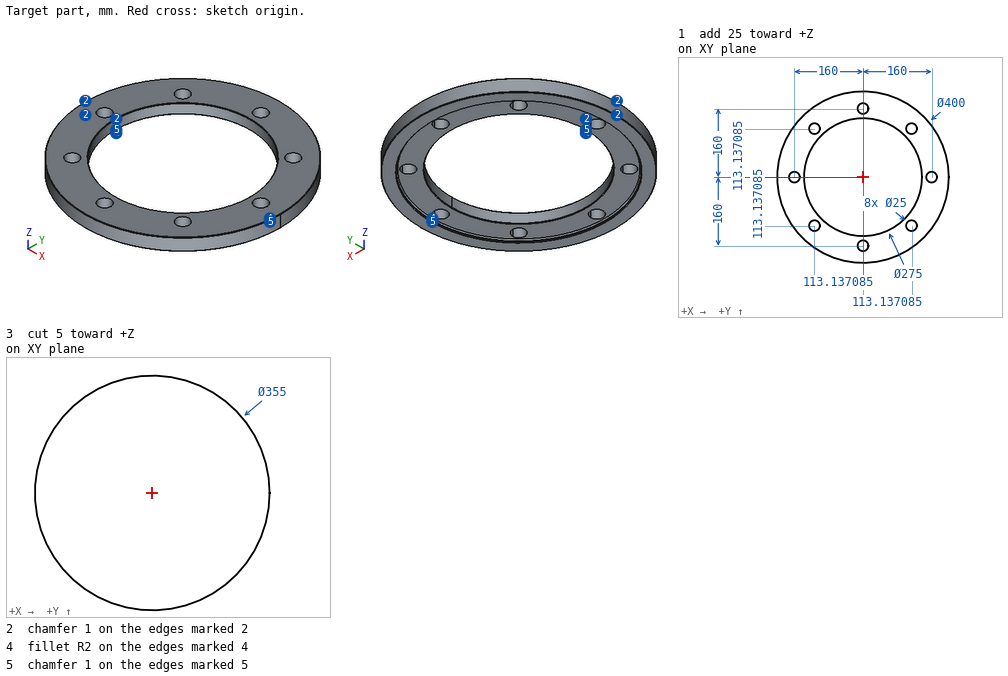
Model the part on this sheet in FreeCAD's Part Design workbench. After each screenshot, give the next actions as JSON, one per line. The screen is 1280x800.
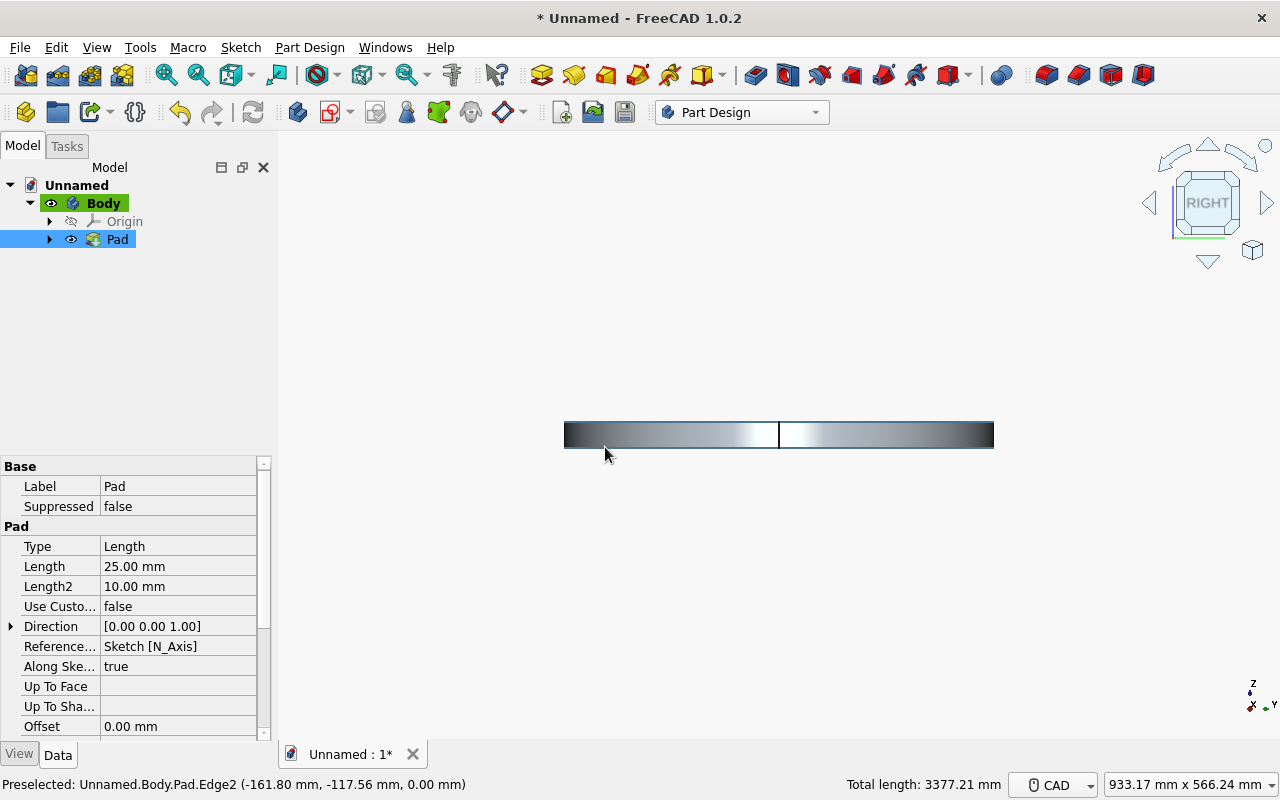
{"action": "left_click", "coordinate": [168, 76]}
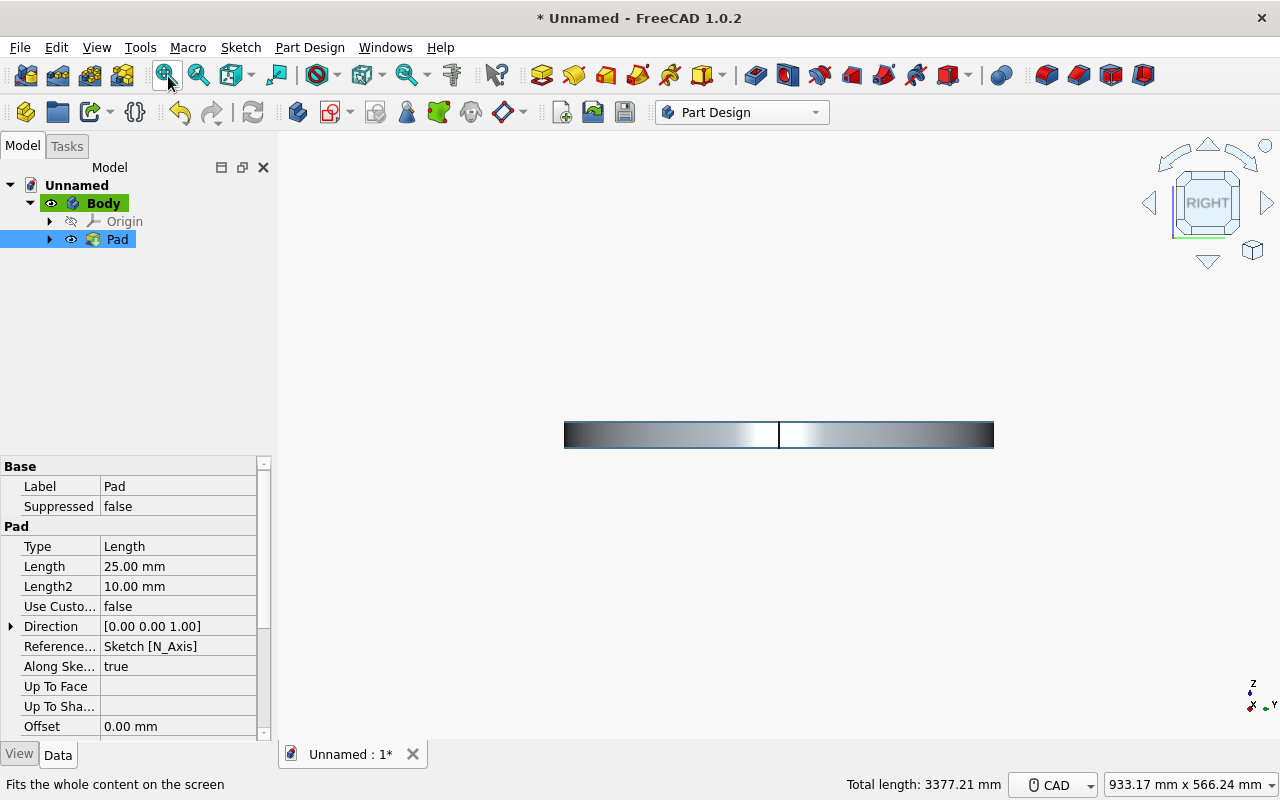
{"action": "key", "text": "5"}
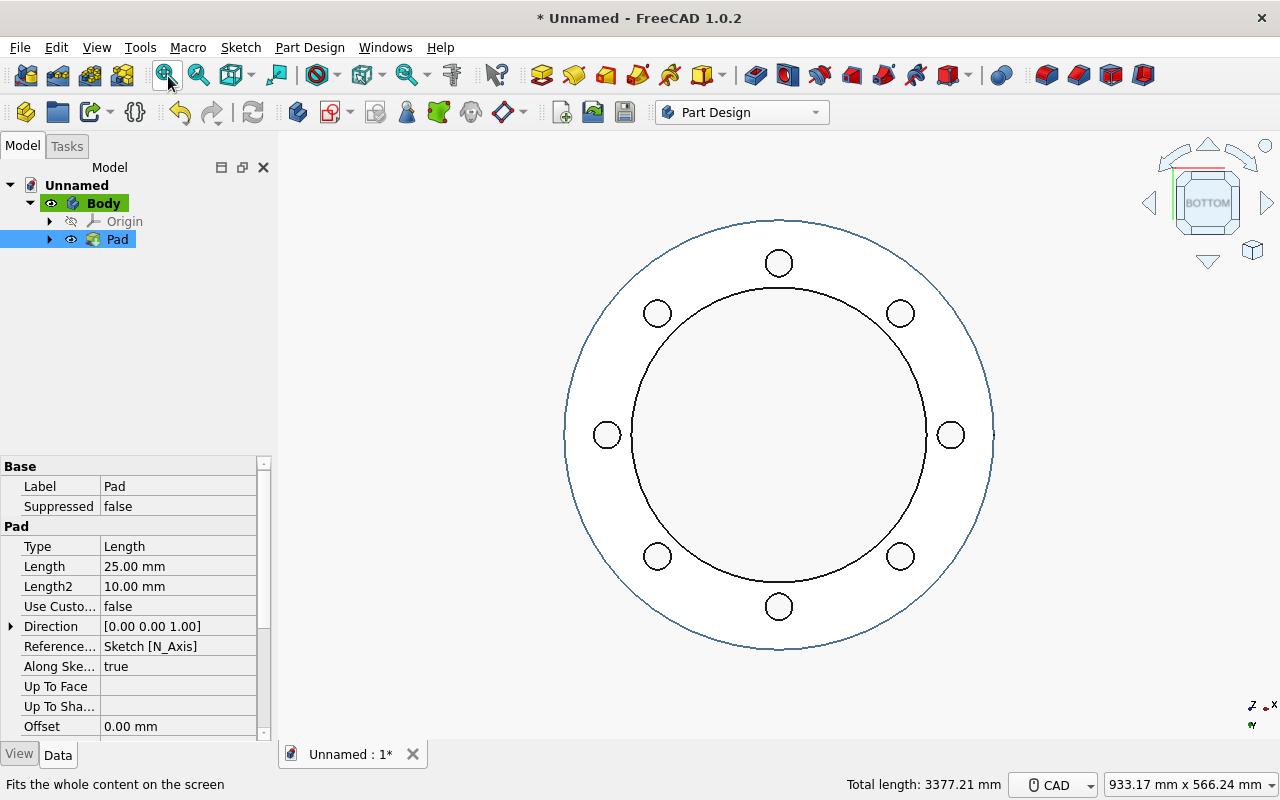
{"action": "left_click", "coordinate": [631, 434], "text": "ctrl"}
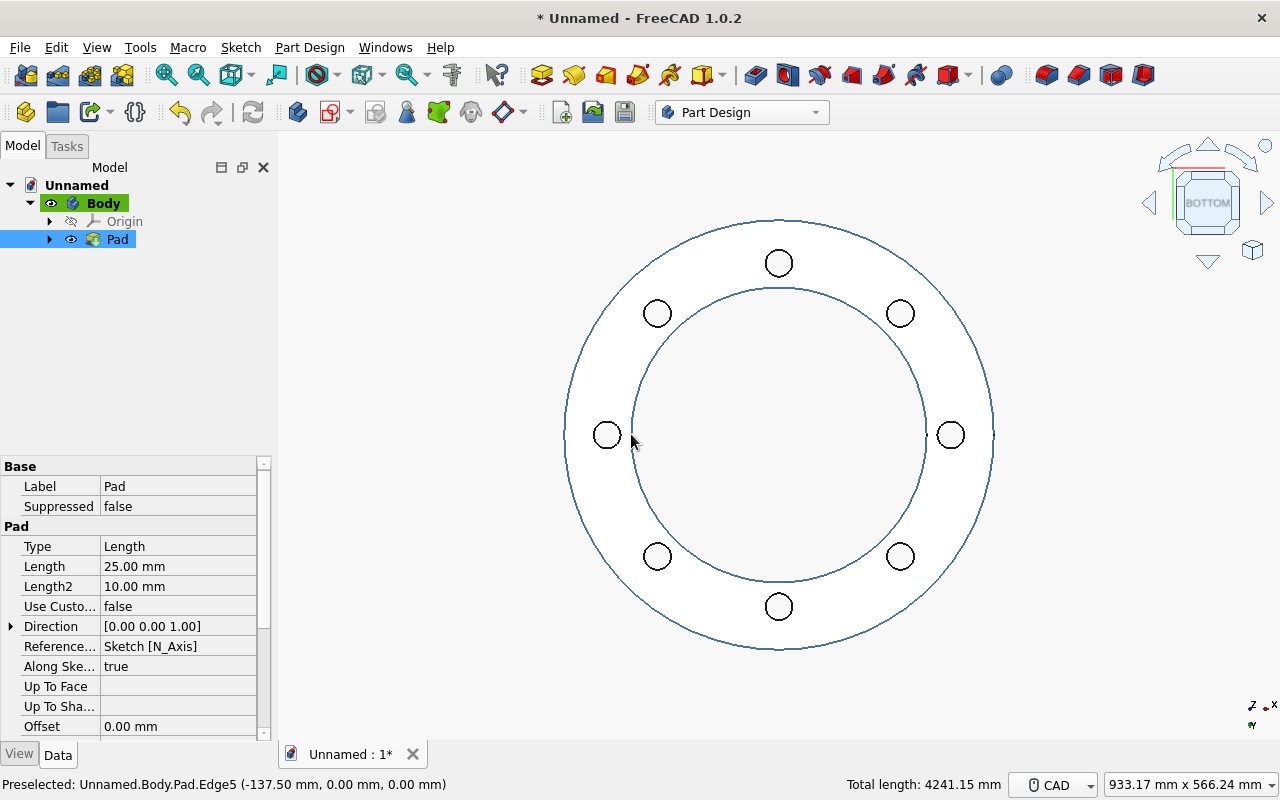
{"action": "left_click", "coordinate": [1080, 76]}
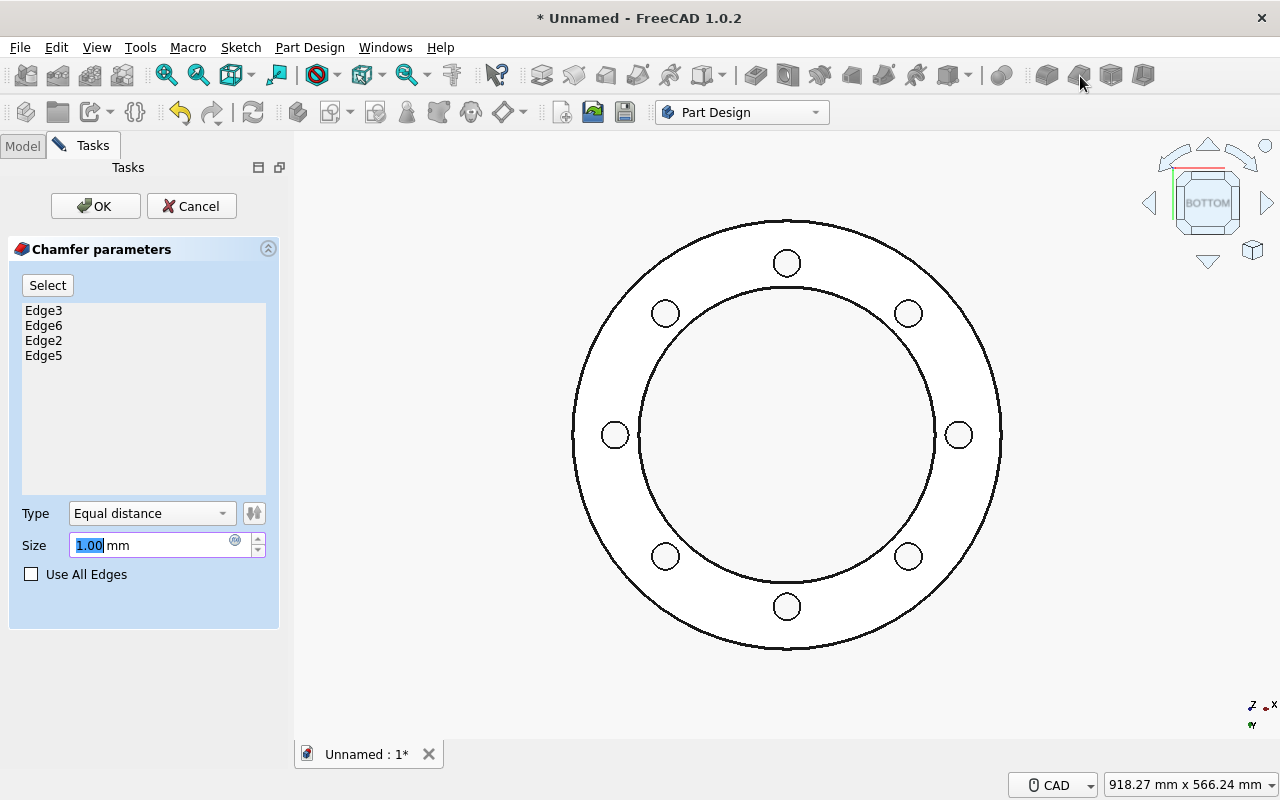
{"action": "type", "text": "1"}
{"action": "key", "text": "Tab"}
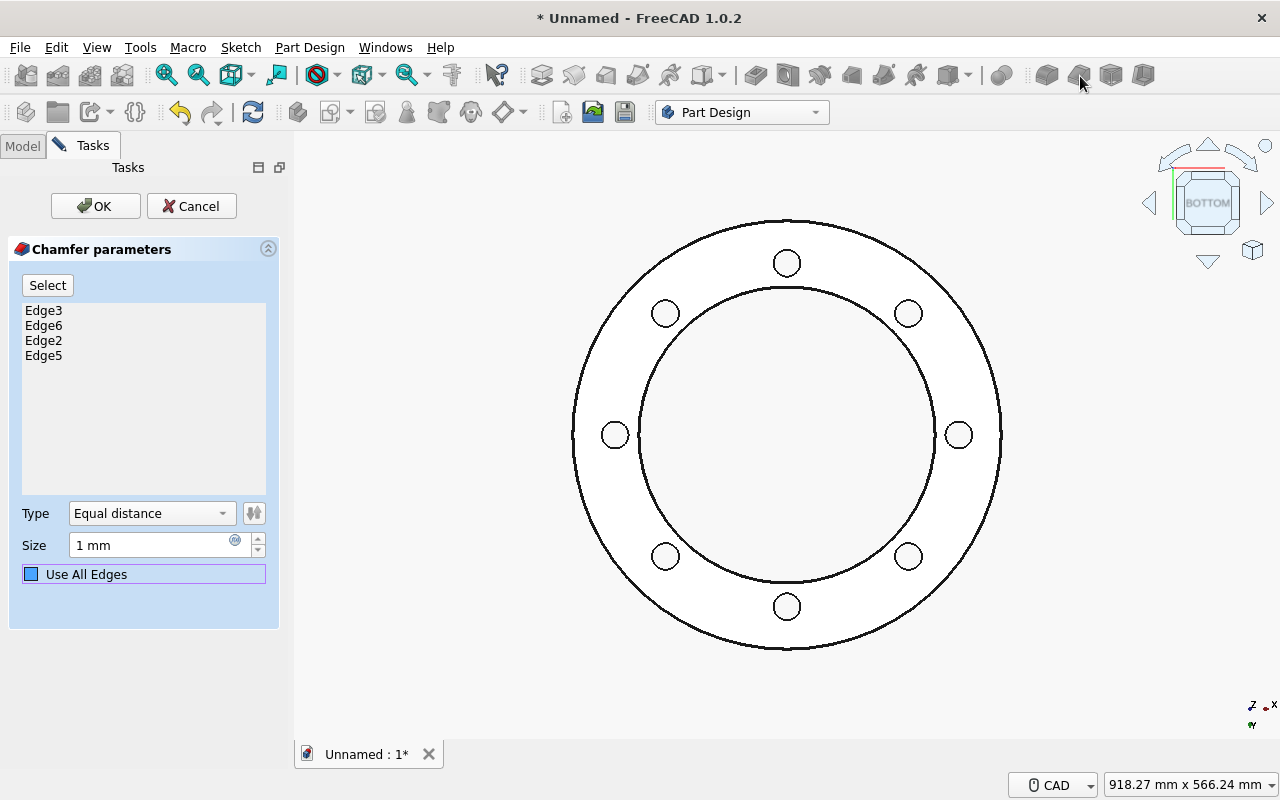
{"action": "left_click", "coordinate": [96, 206]}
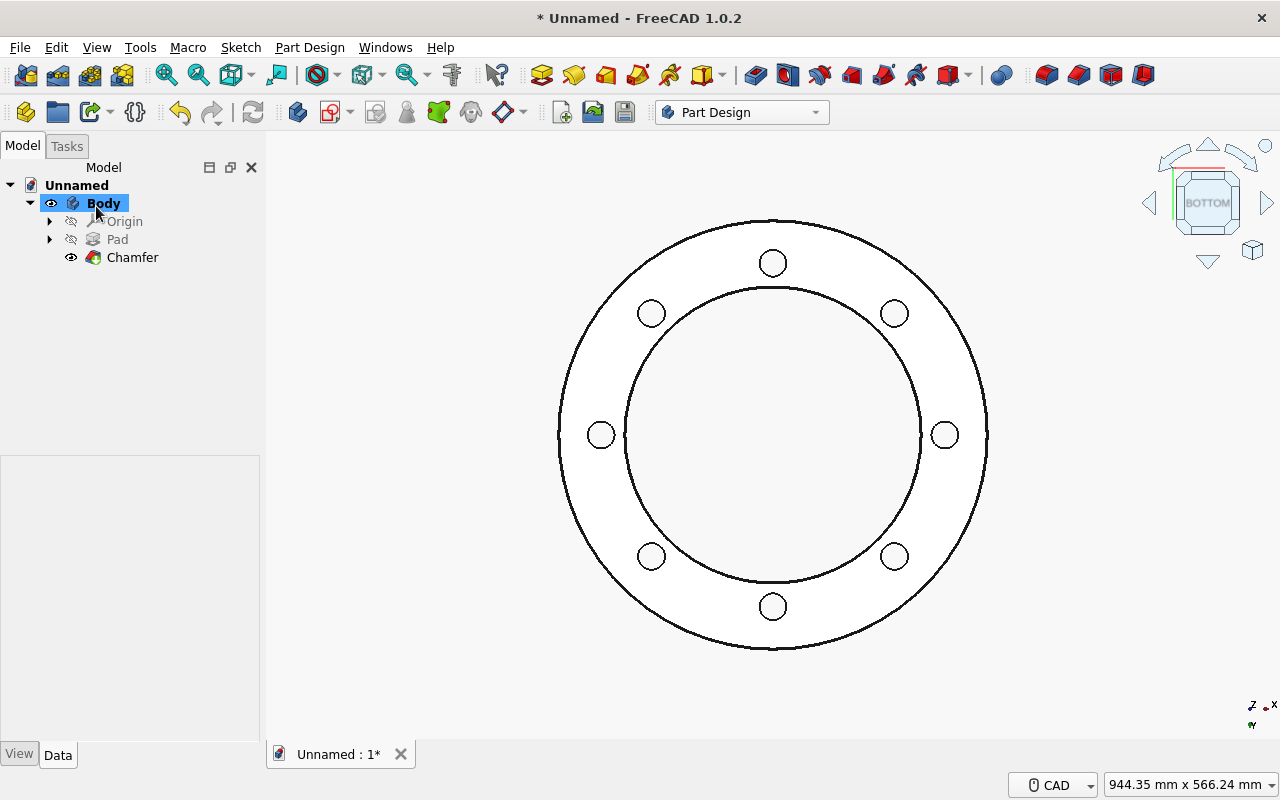
{"action": "left_click", "coordinate": [330, 112]}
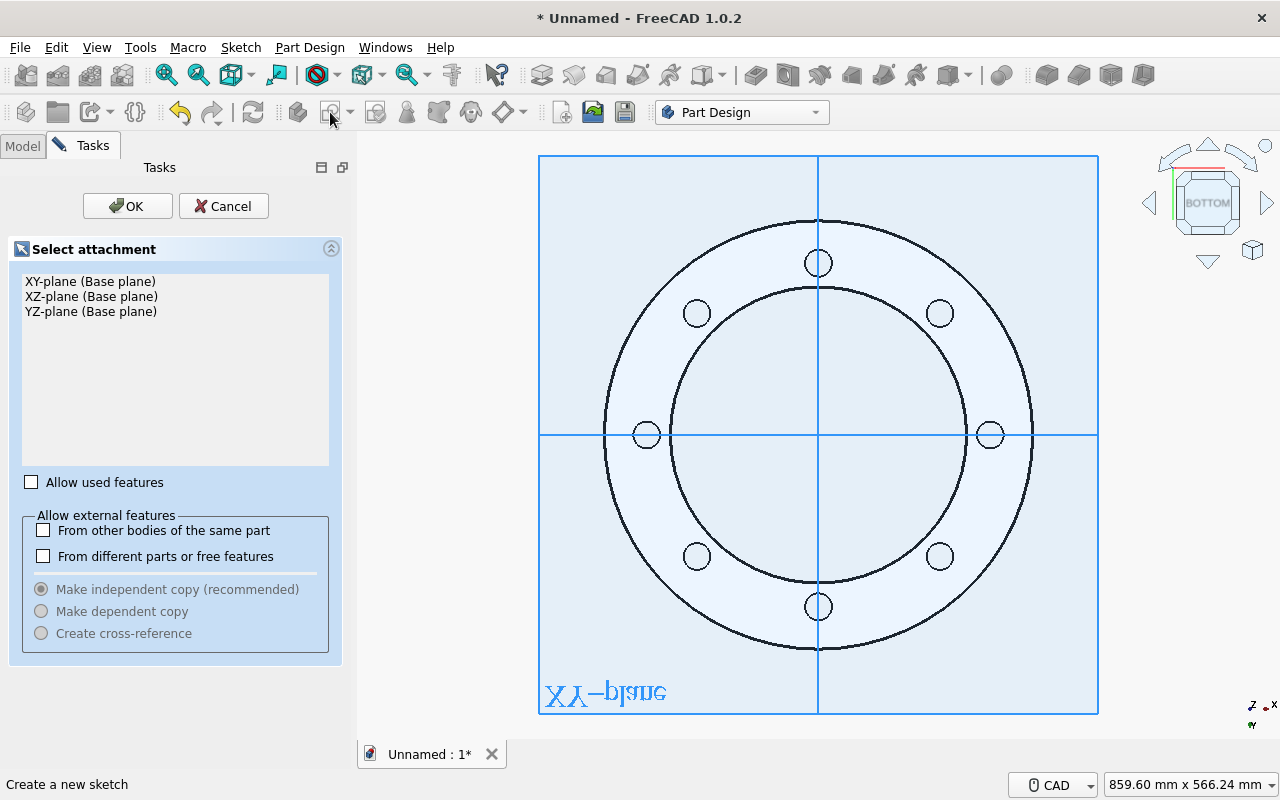
{"action": "left_click", "coordinate": [82, 282]}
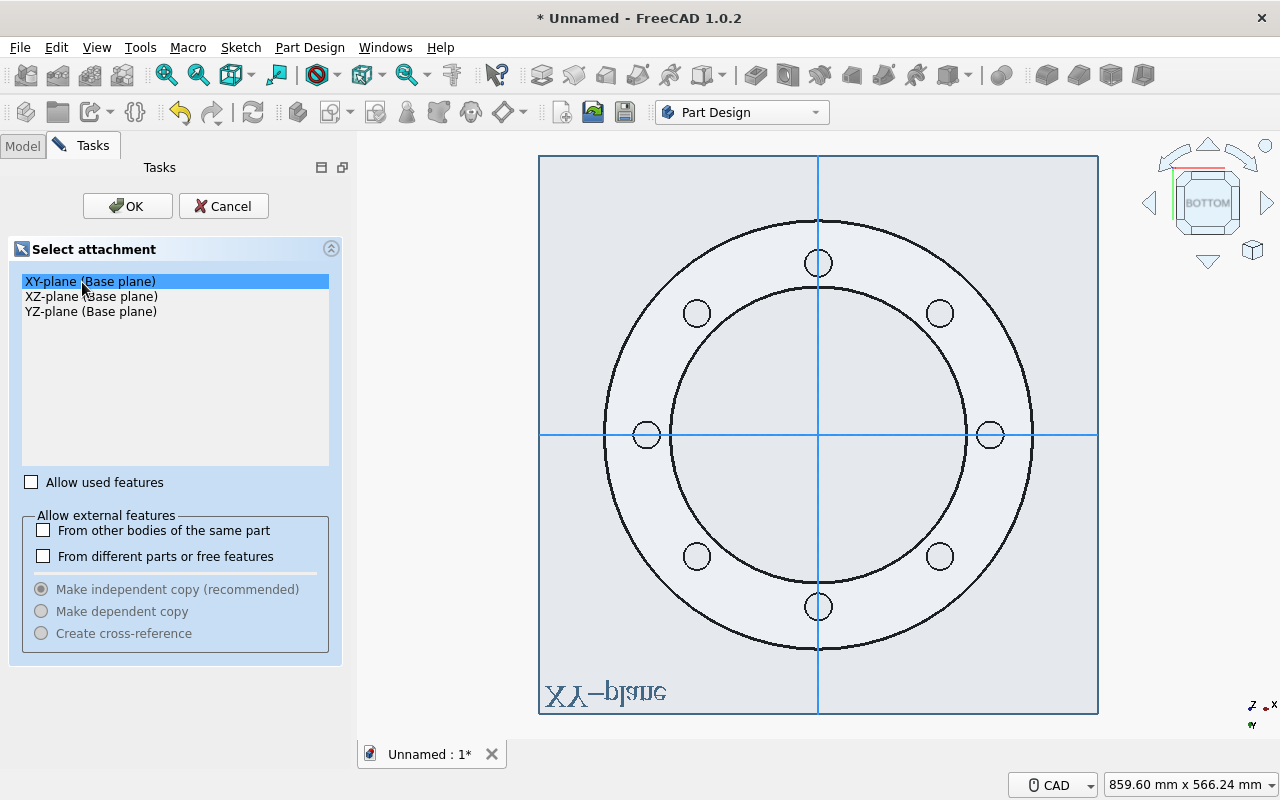
{"action": "left_click", "coordinate": [128, 206]}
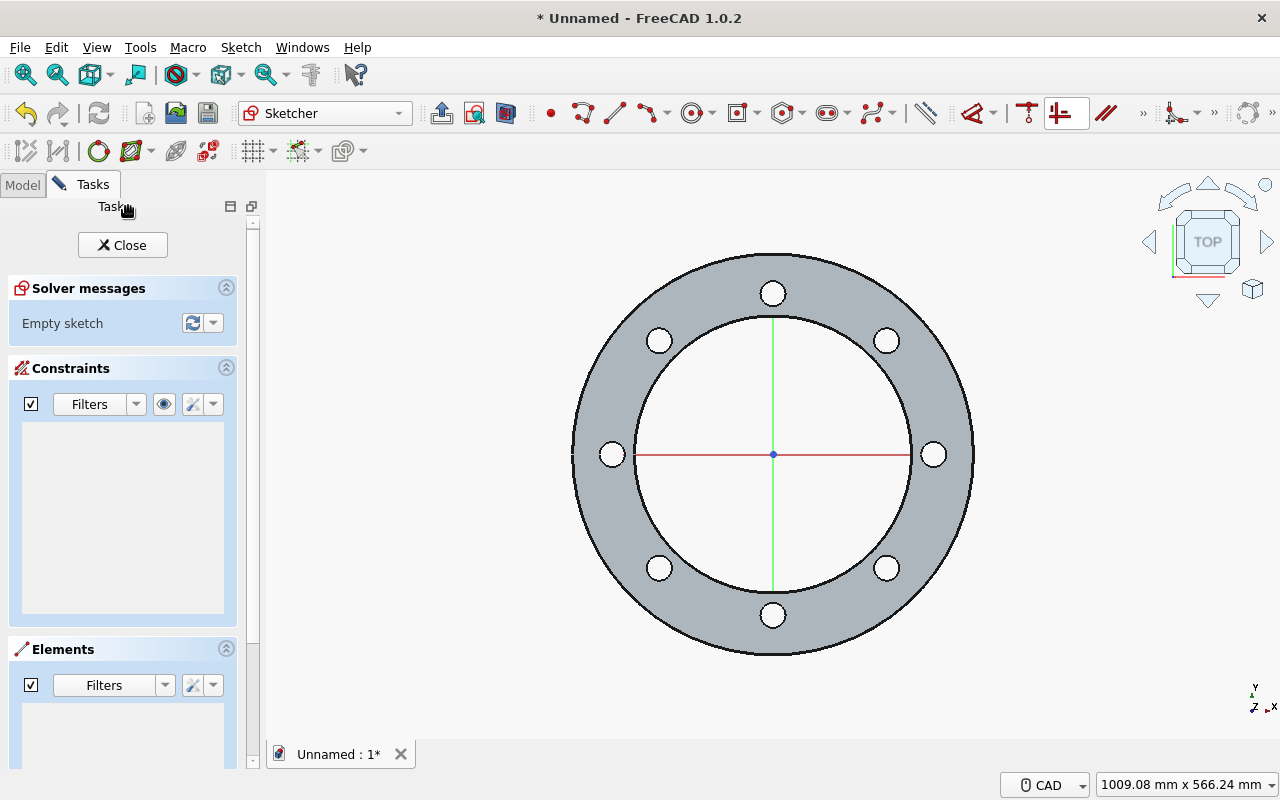
{"action": "left_click", "coordinate": [506, 114]}